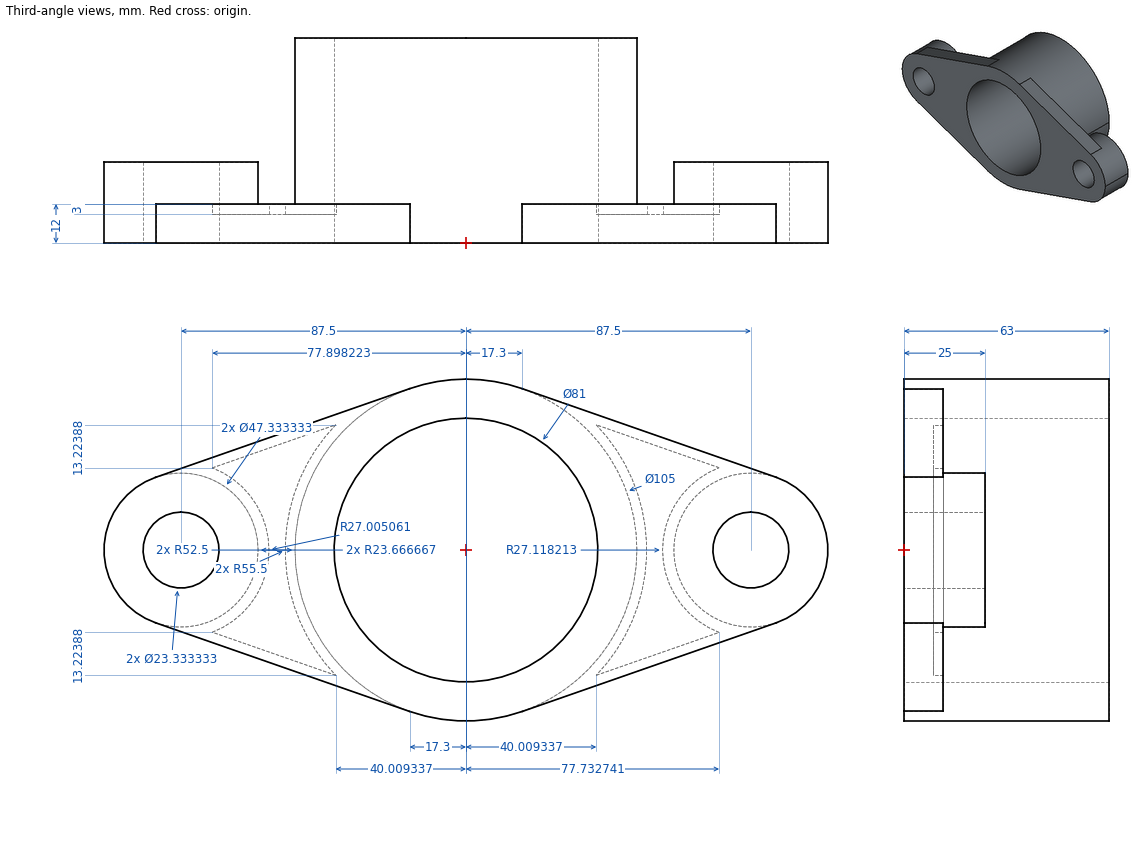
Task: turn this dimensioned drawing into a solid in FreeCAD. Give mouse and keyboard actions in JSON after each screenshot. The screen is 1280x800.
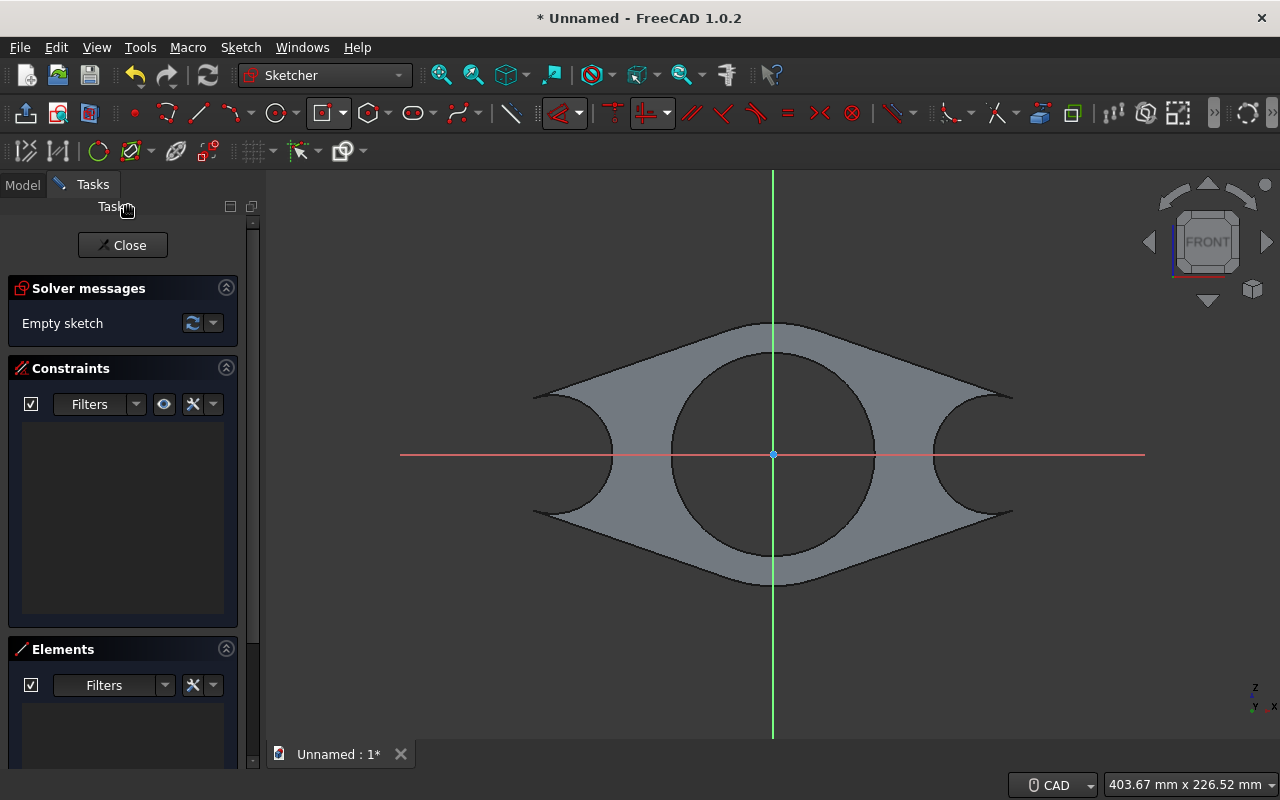
{"action": "key", "text": "g c"}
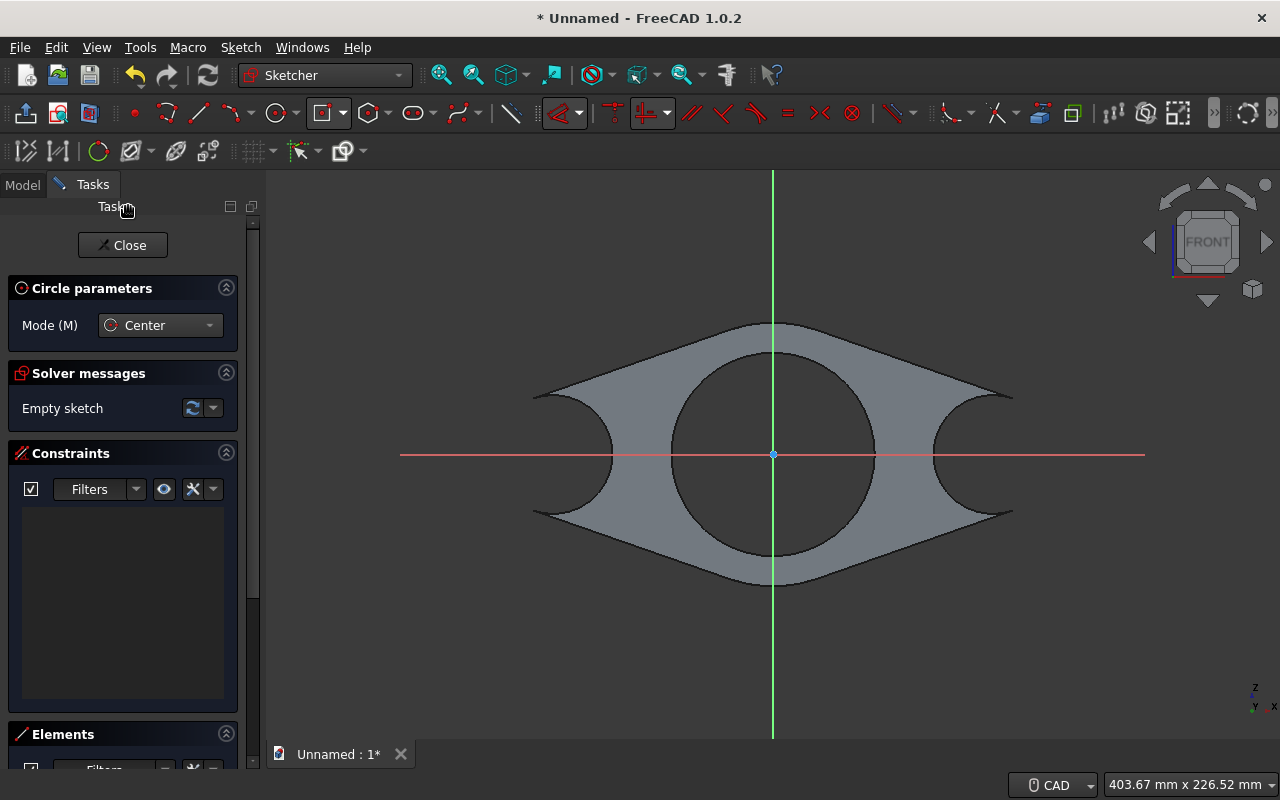
{"action": "left_click", "coordinate": [553, 455]}
{"action": "left_click", "coordinate": [595, 412]}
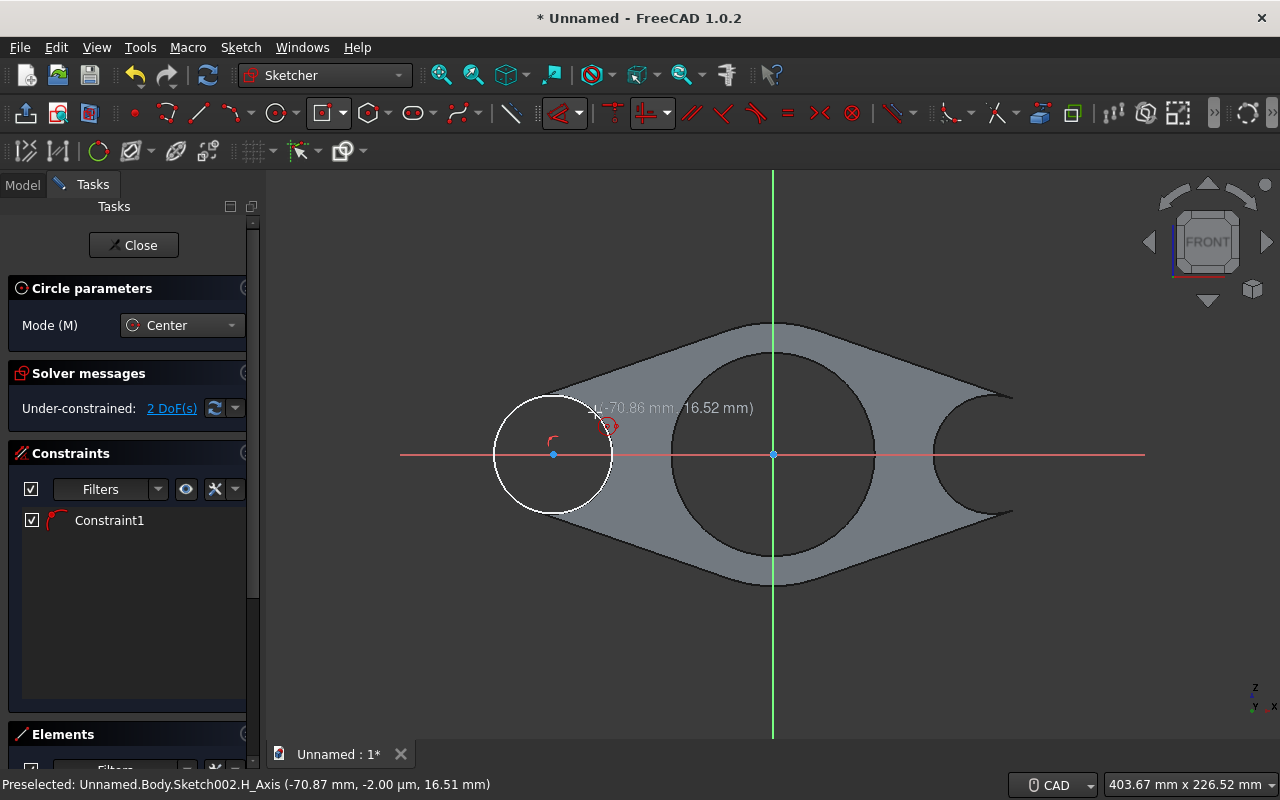
{"action": "left_click", "coordinate": [993, 455]}
{"action": "left_click", "coordinate": [1035, 412]}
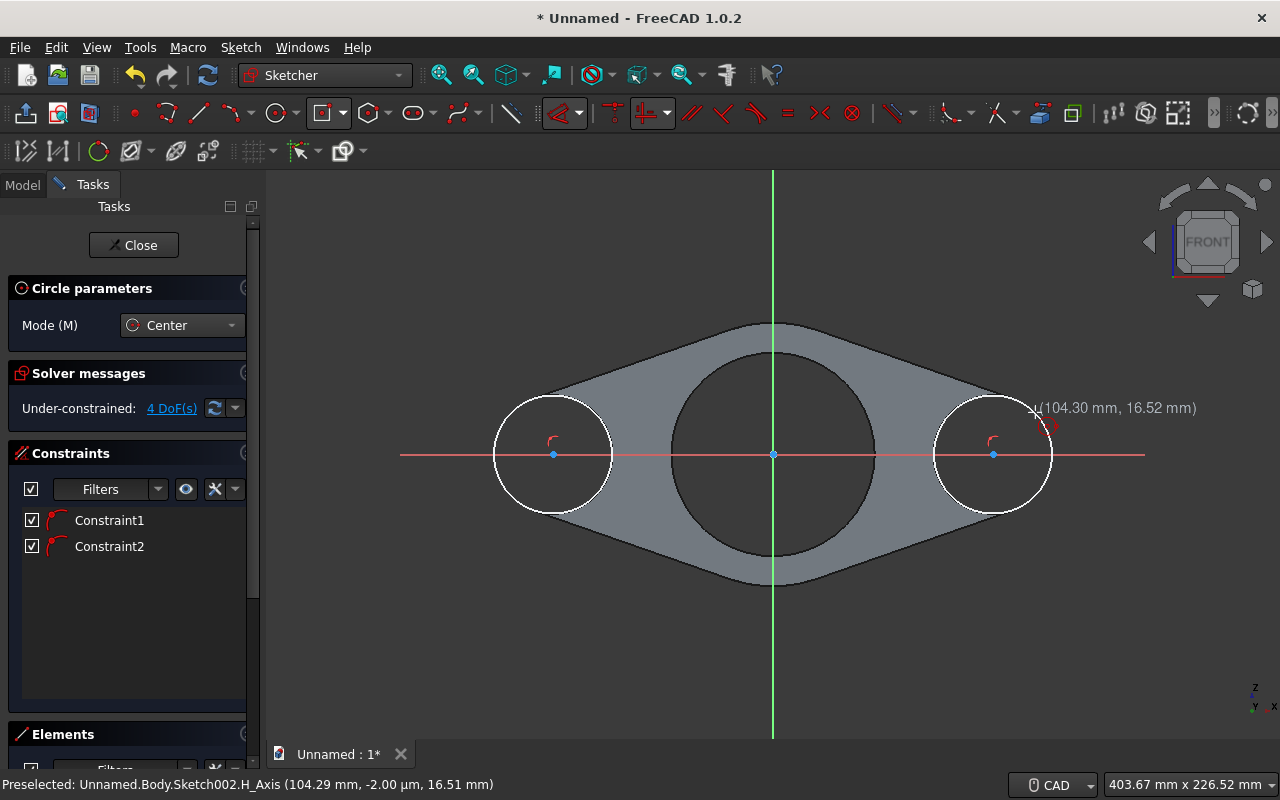
{"action": "left_click", "coordinate": [553, 455]}
{"action": "left_click", "coordinate": [574, 434]}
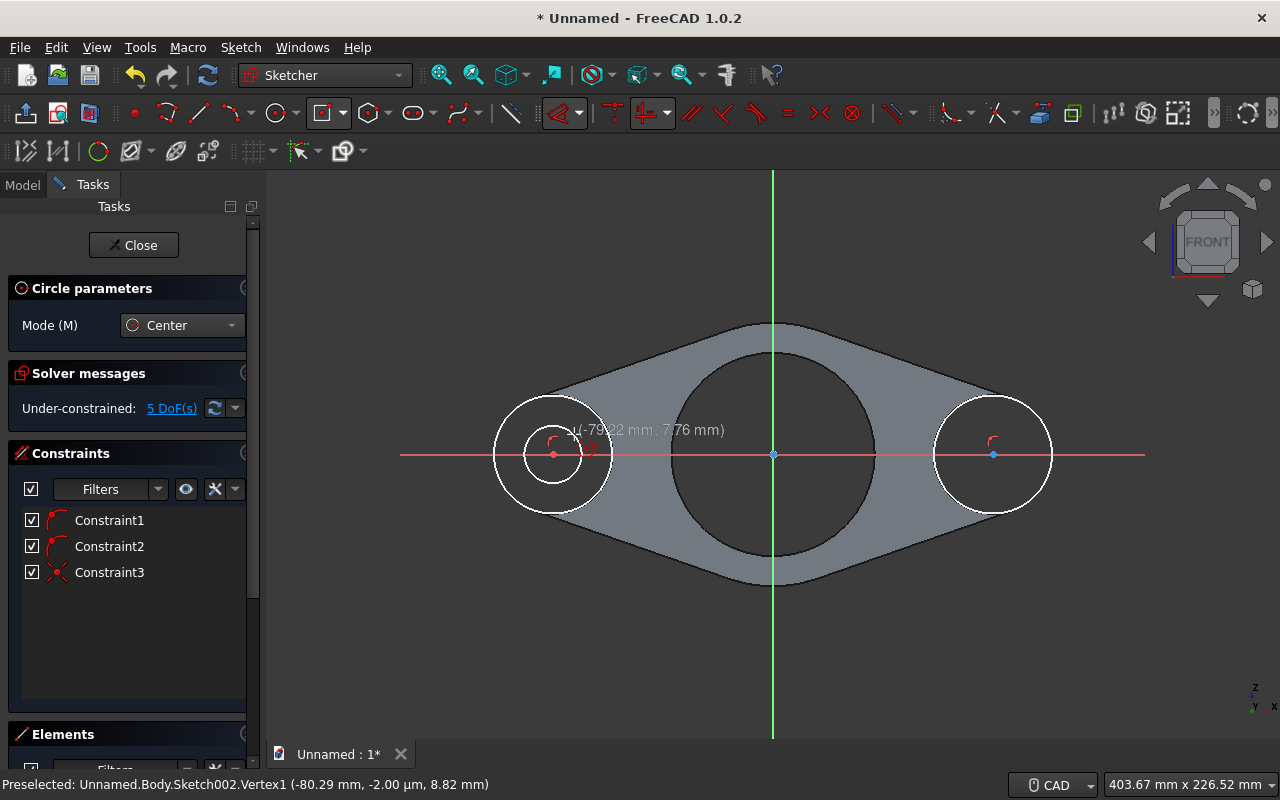
{"action": "left_click", "coordinate": [993, 455]}
{"action": "left_click", "coordinate": [1014, 434]}
{"action": "key", "text": "Escape"}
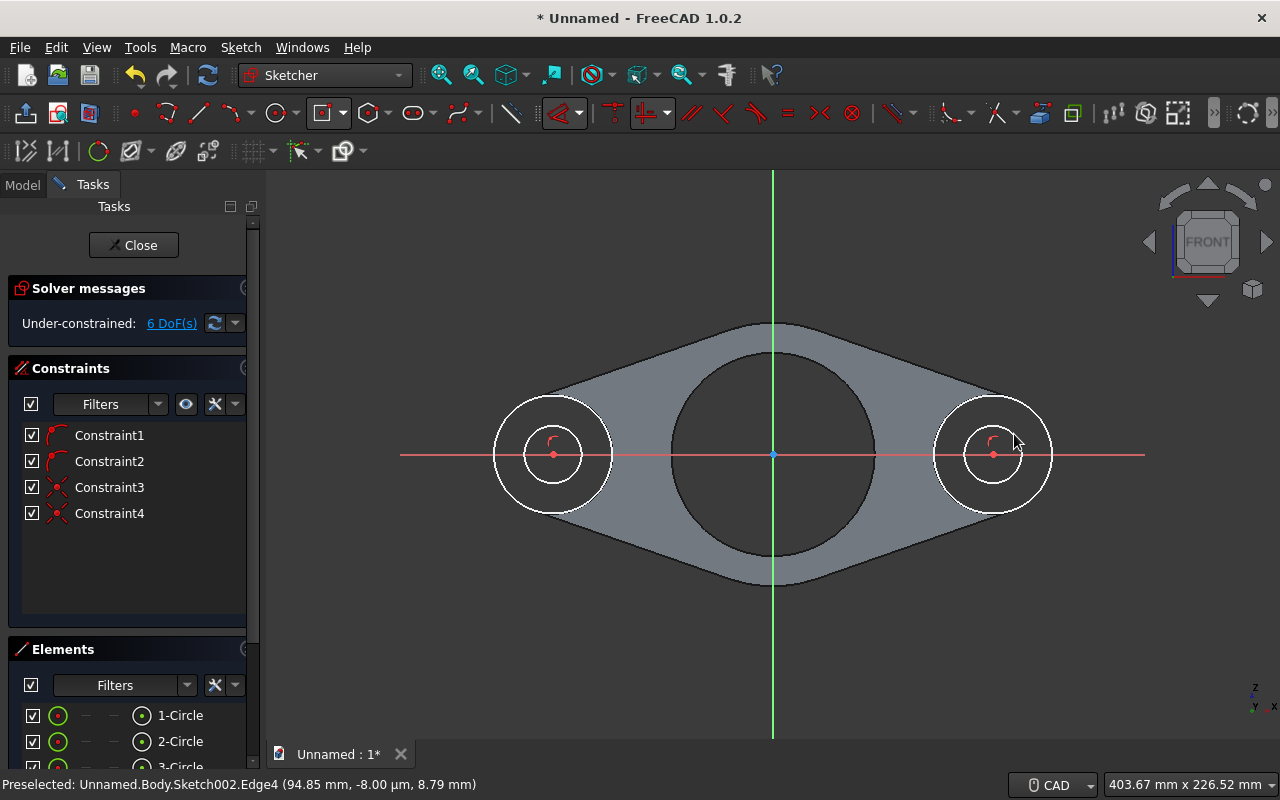
{"action": "left_click", "coordinate": [595, 413]}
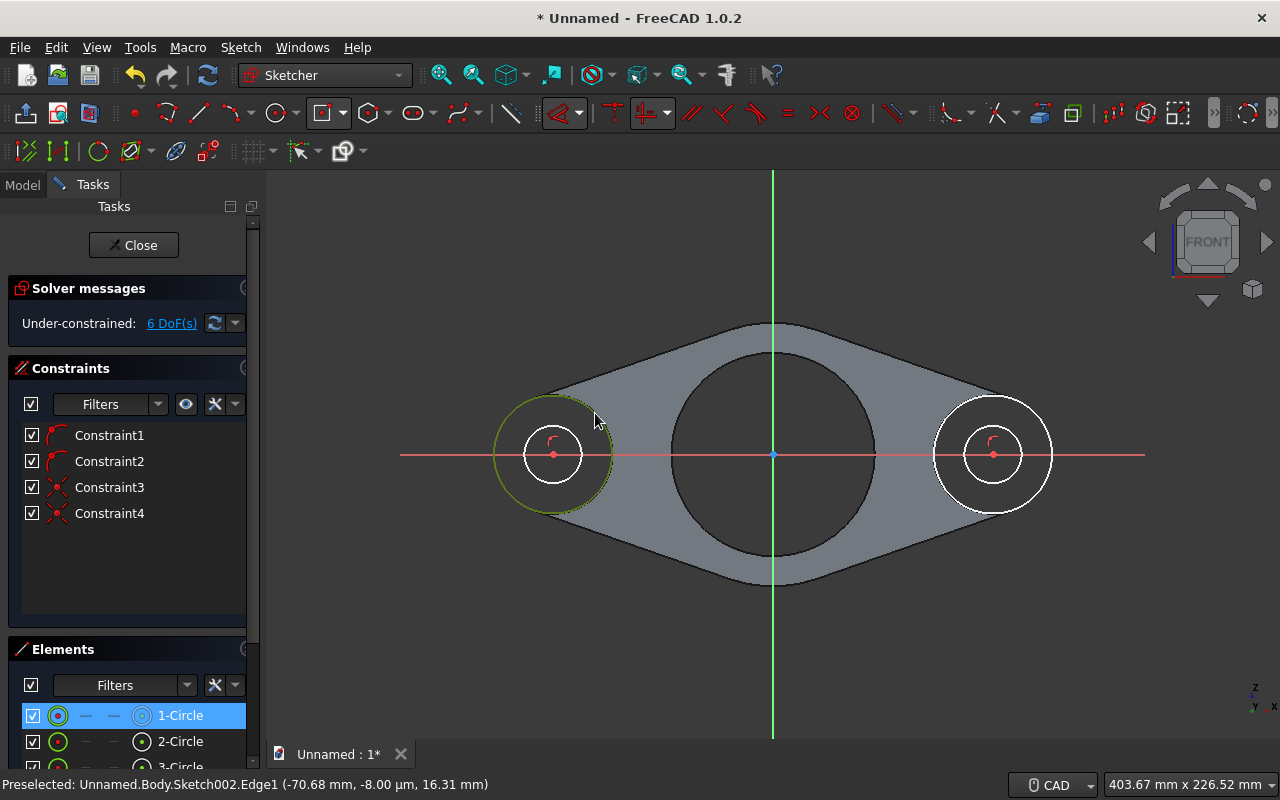
{"action": "left_click", "coordinate": [1035, 413]}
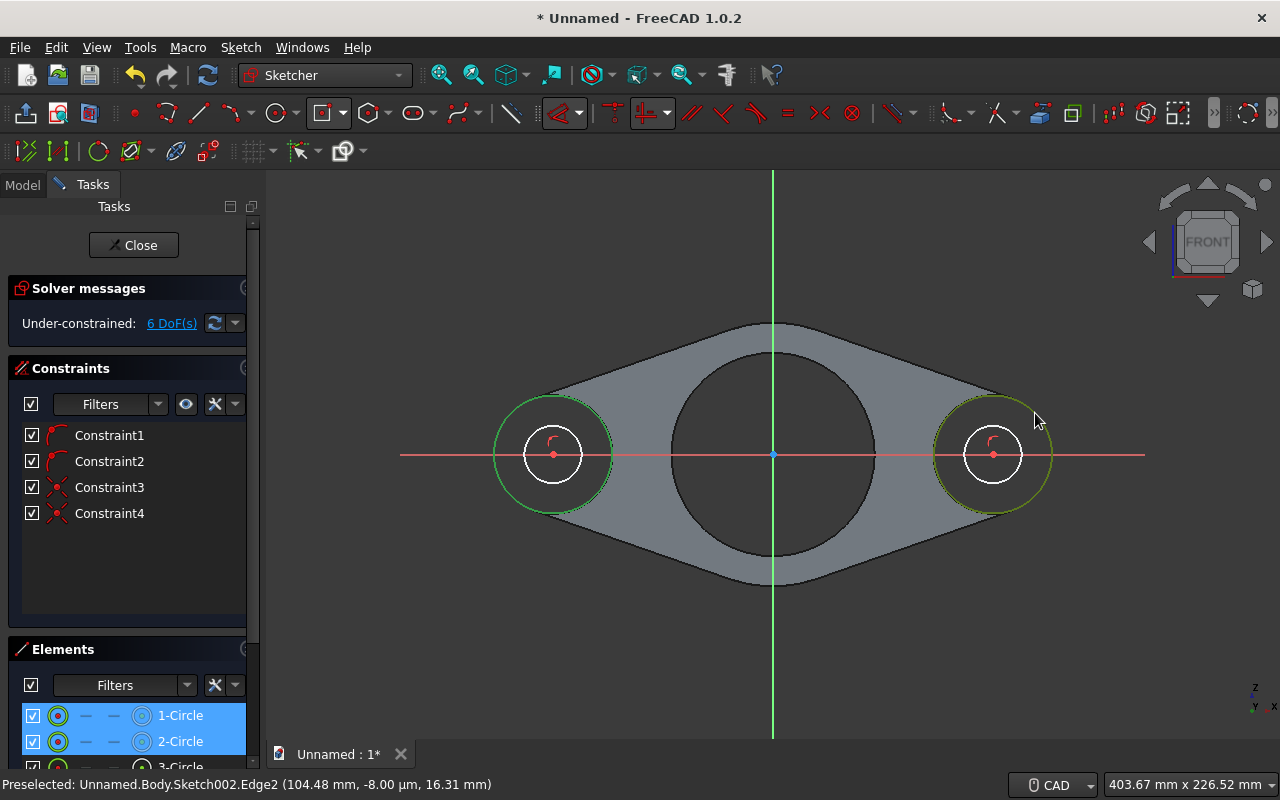
{"action": "key", "text": "e"}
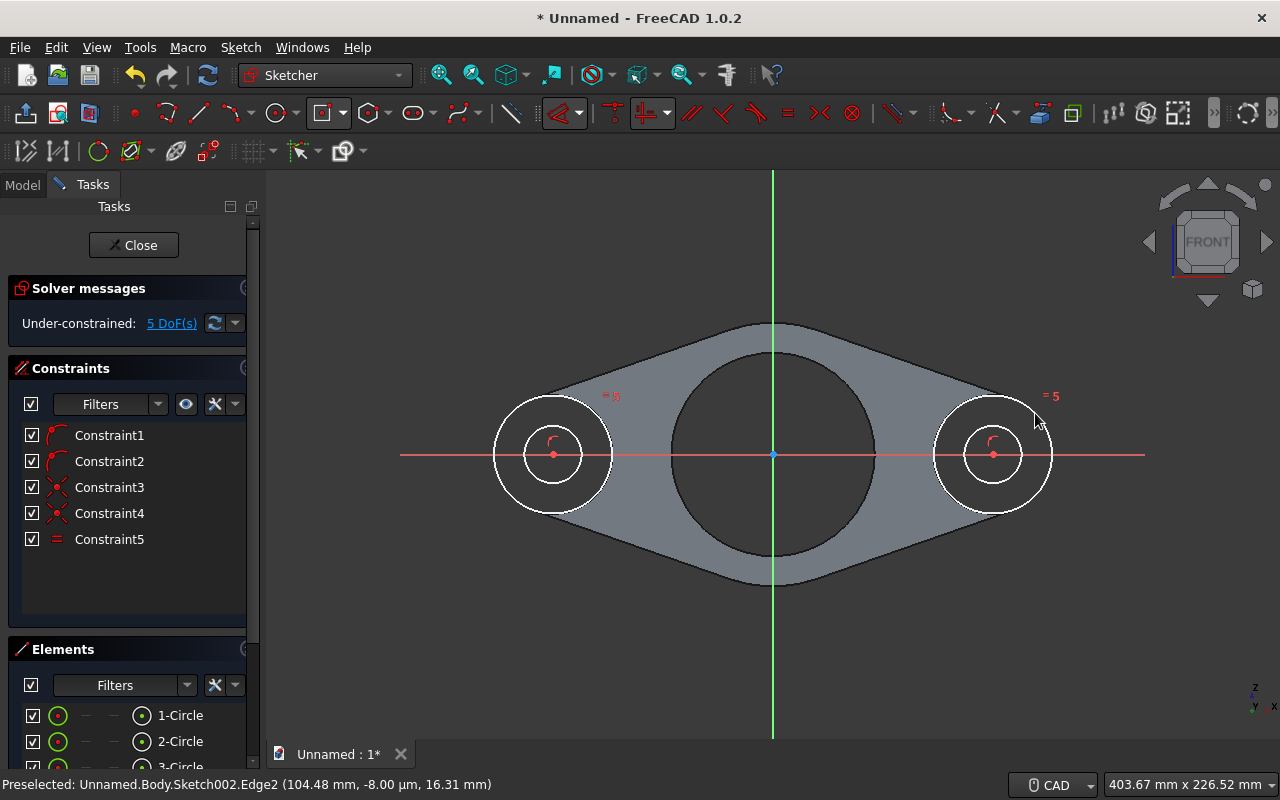
{"action": "left_click", "coordinate": [573, 434]}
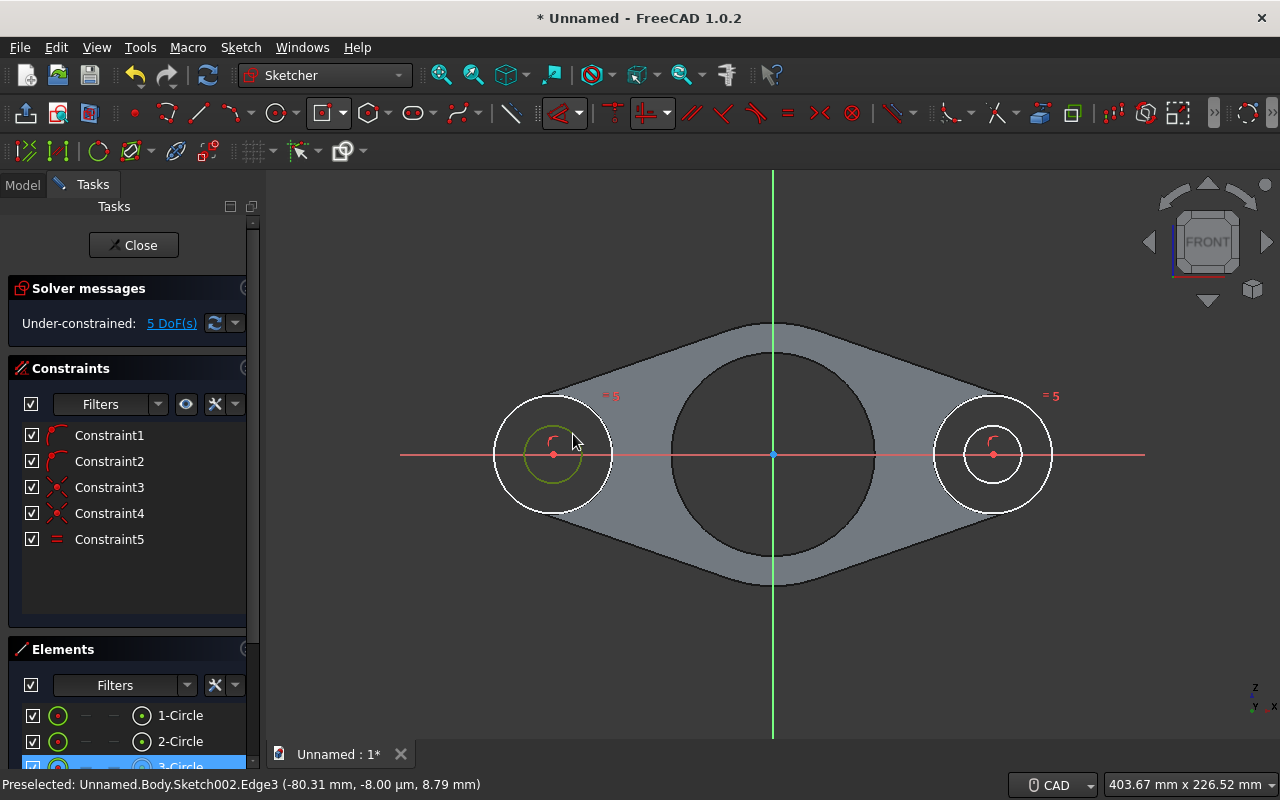
{"action": "left_click", "coordinate": [1013, 434]}